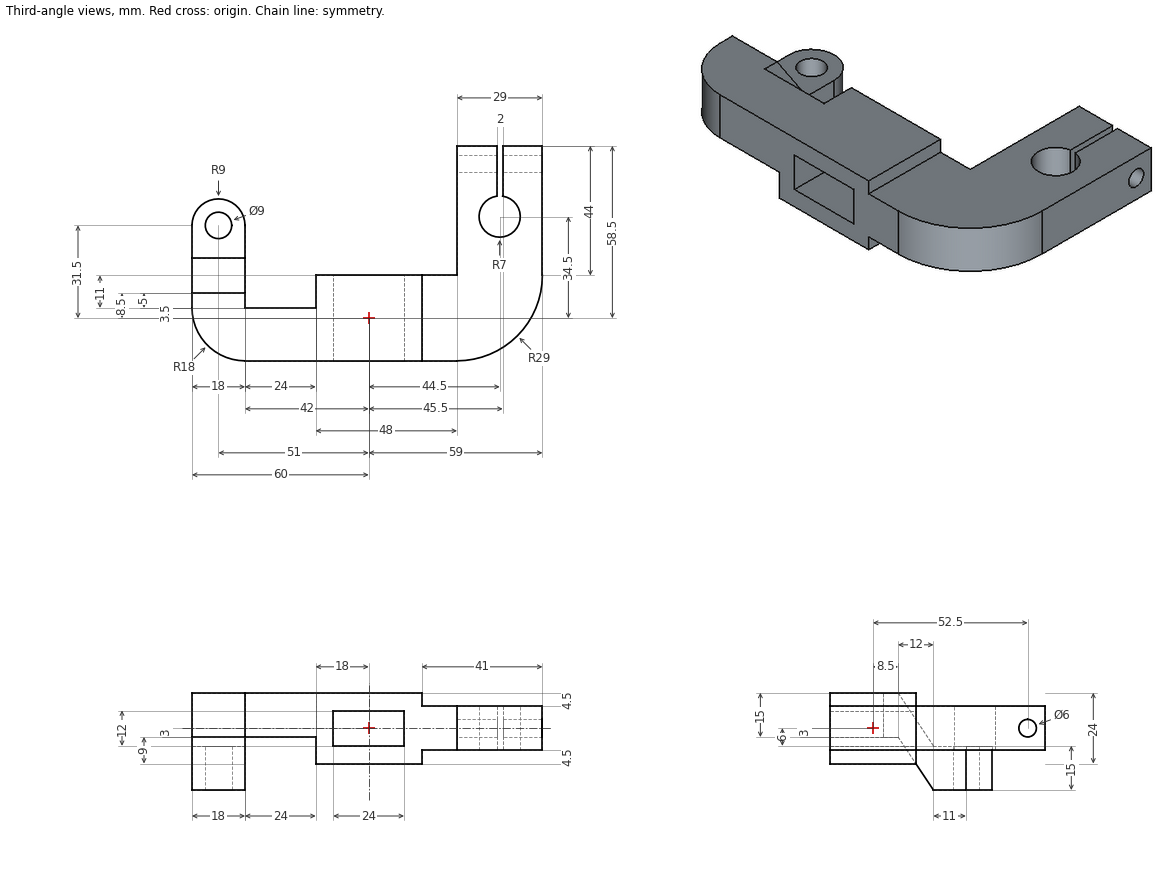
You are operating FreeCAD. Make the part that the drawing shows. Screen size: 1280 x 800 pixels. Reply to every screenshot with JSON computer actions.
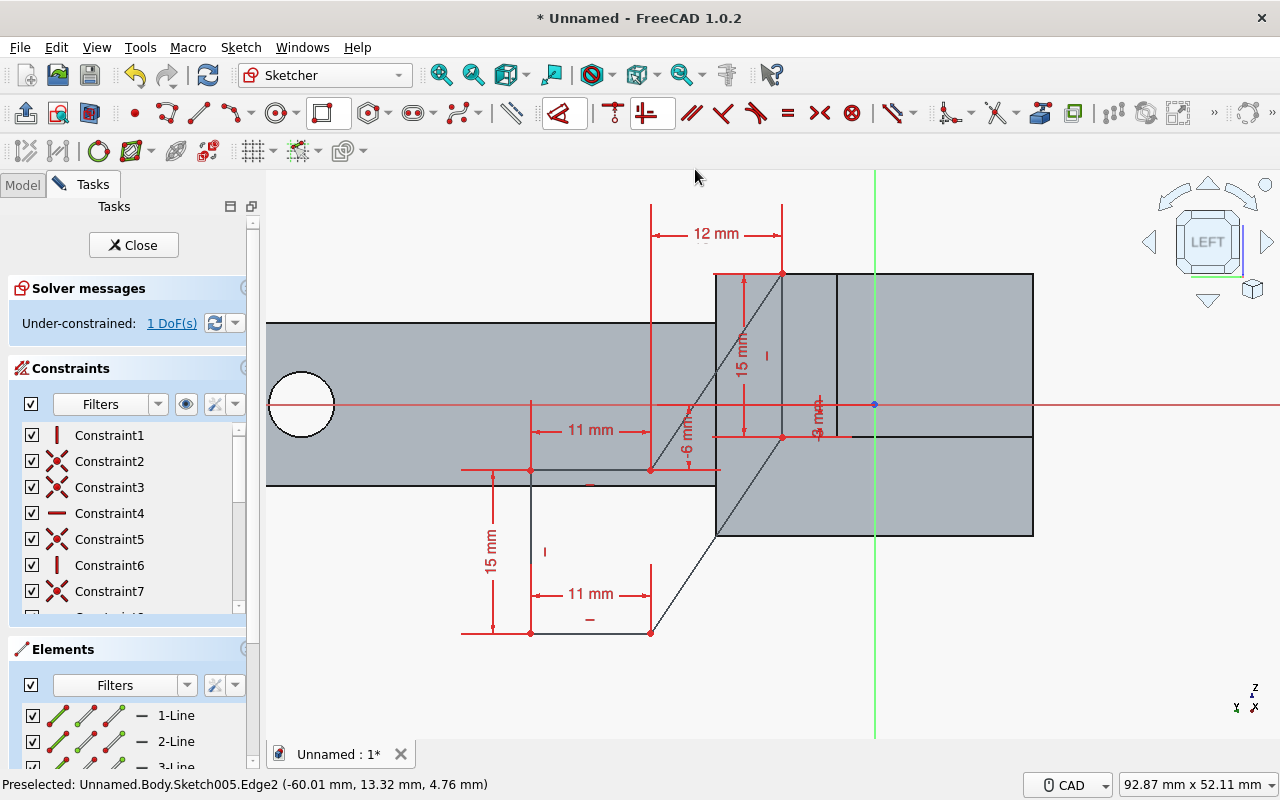
{"action": "left_click", "coordinate": [782, 437]}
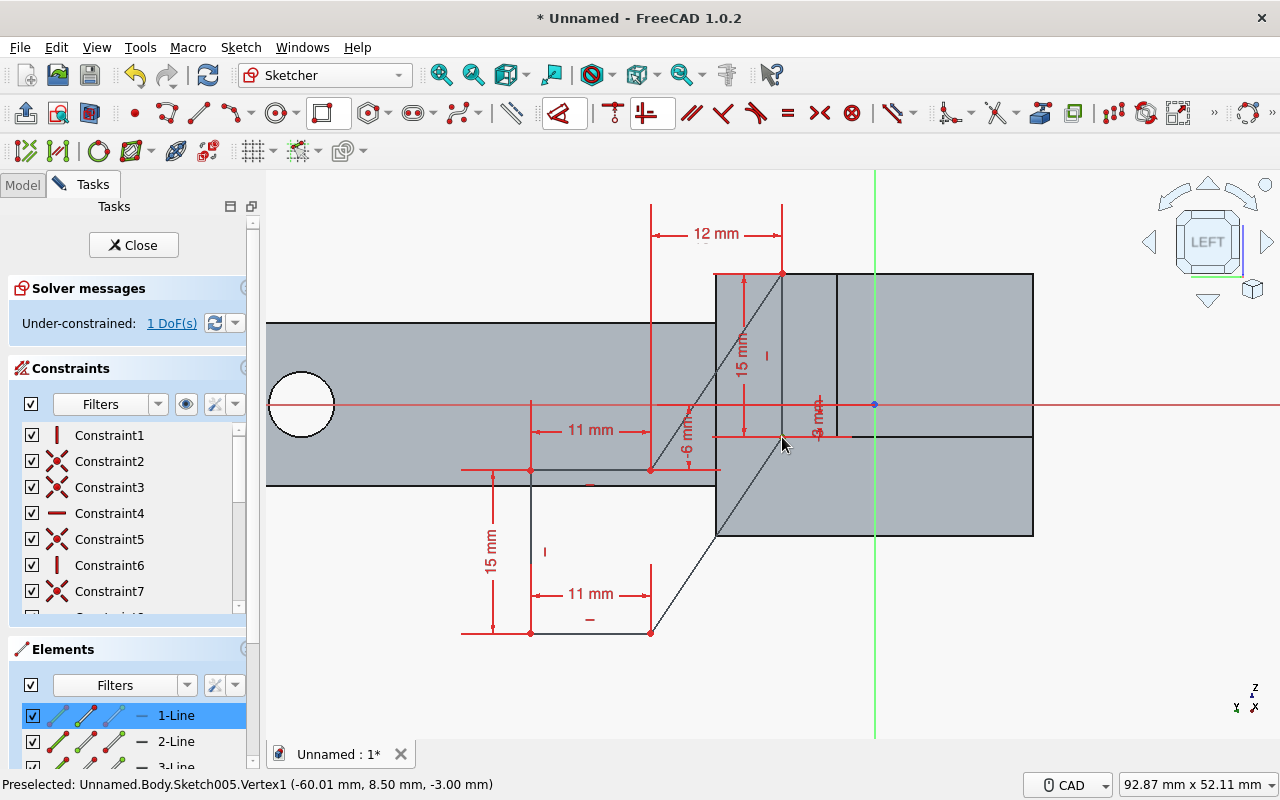
{"action": "left_click", "coordinate": [582, 114]}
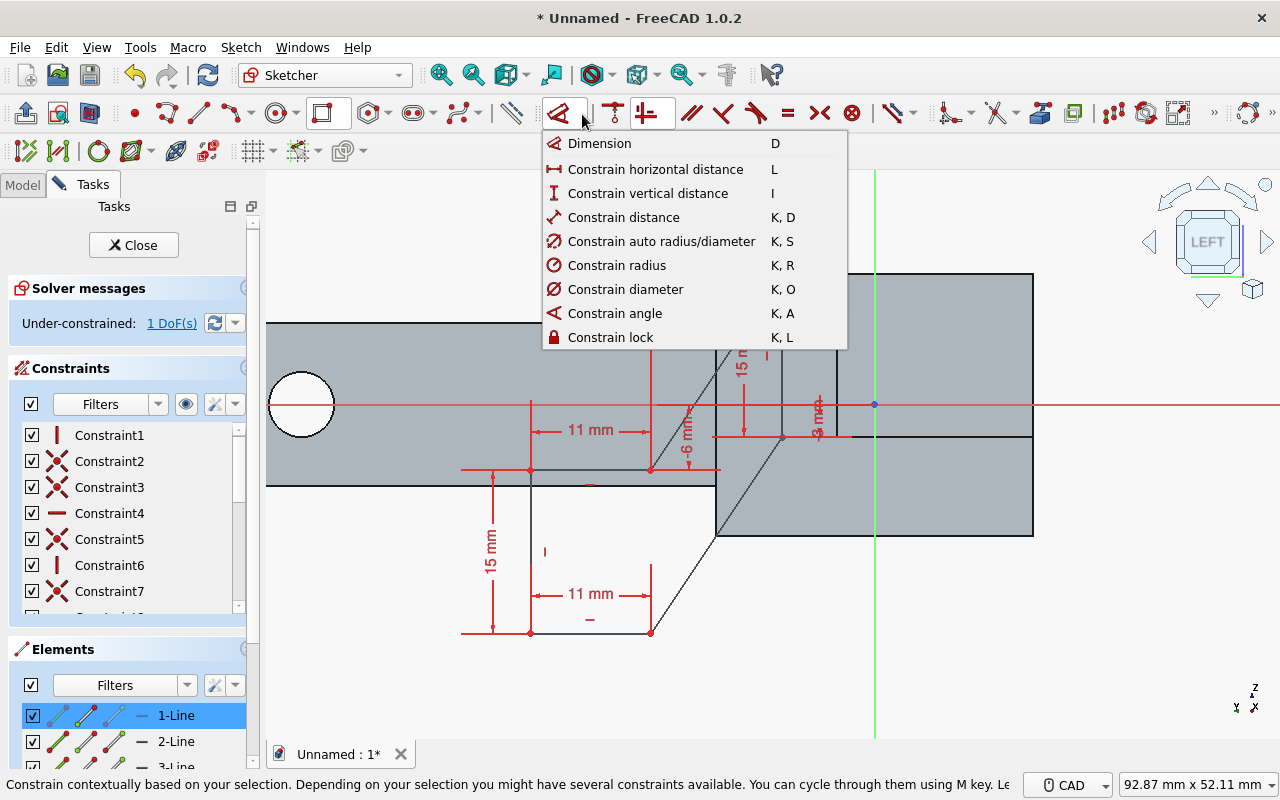
{"action": "left_click", "coordinate": [695, 169]}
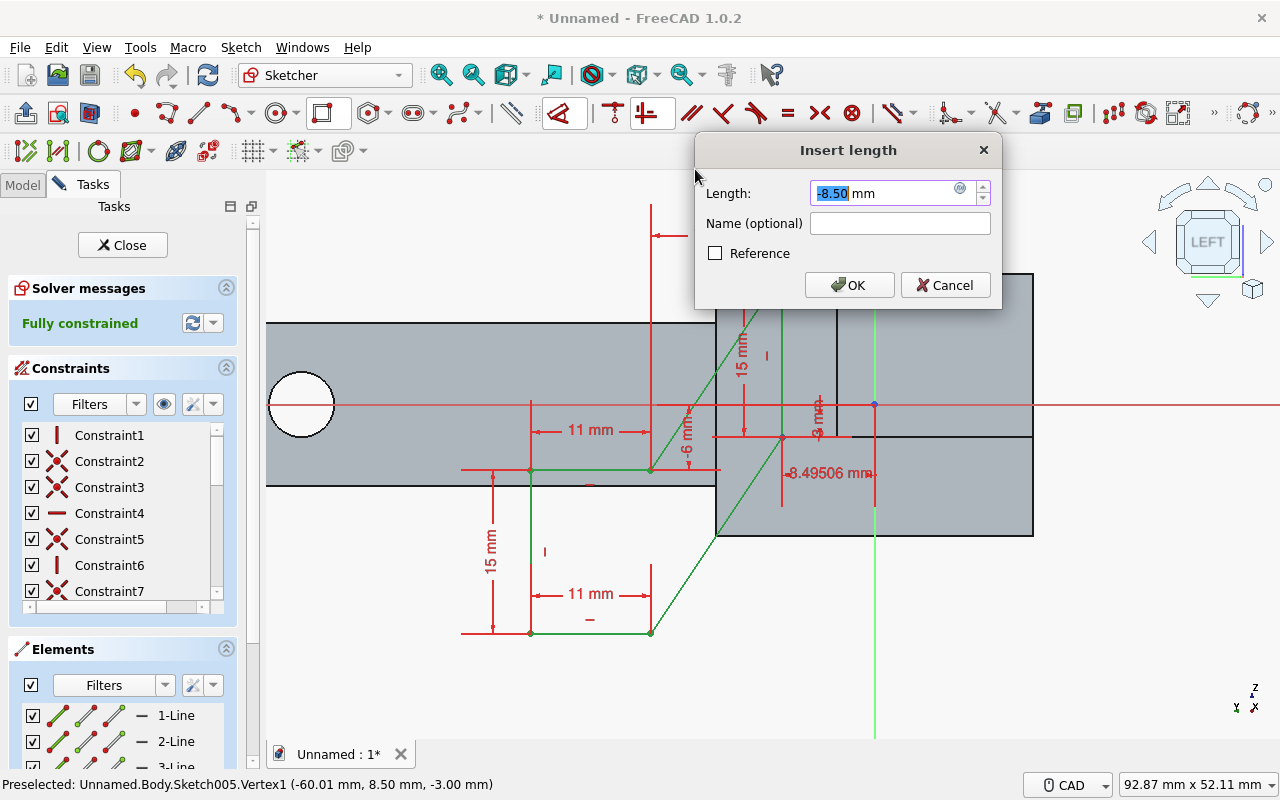
{"action": "type", "text": "-8.5"}
{"action": "key", "text": "Return"}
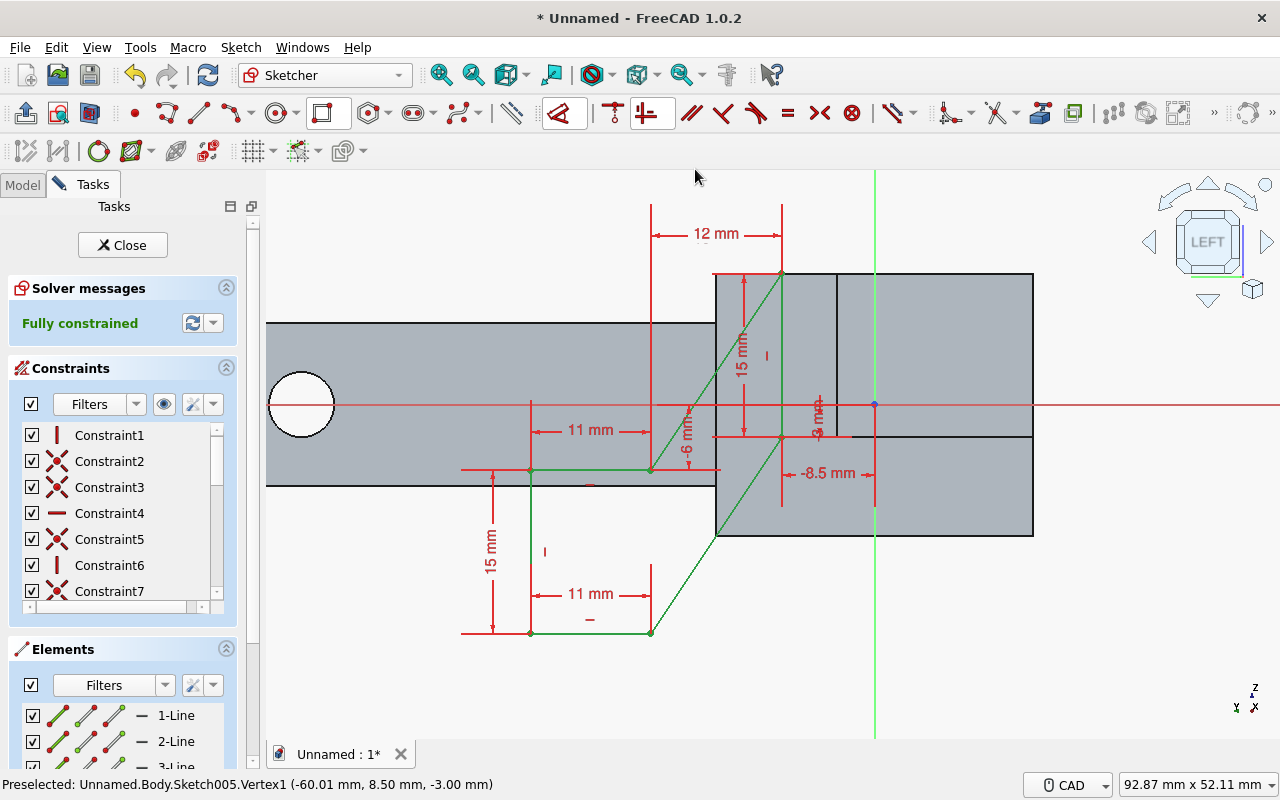
{"action": "left_click", "coordinate": [123, 245]}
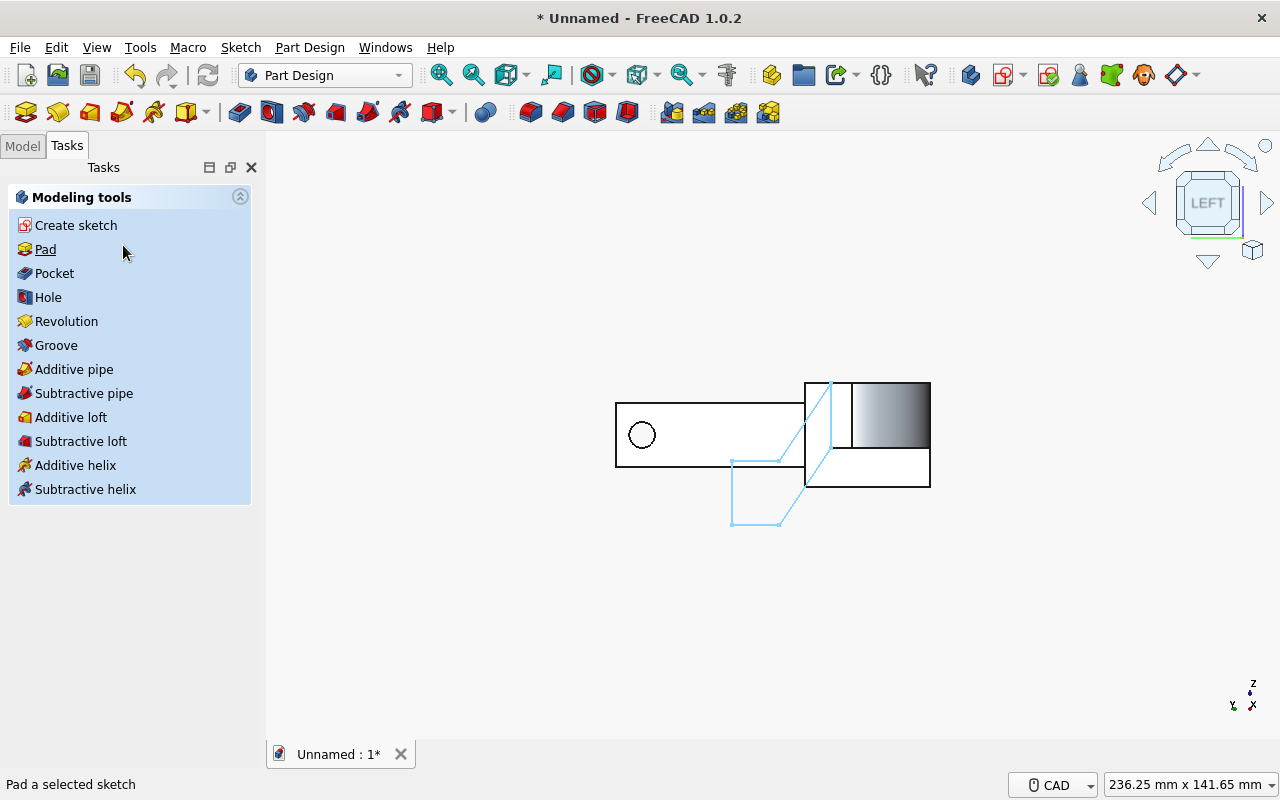
{"action": "left_click", "coordinate": [26, 112]}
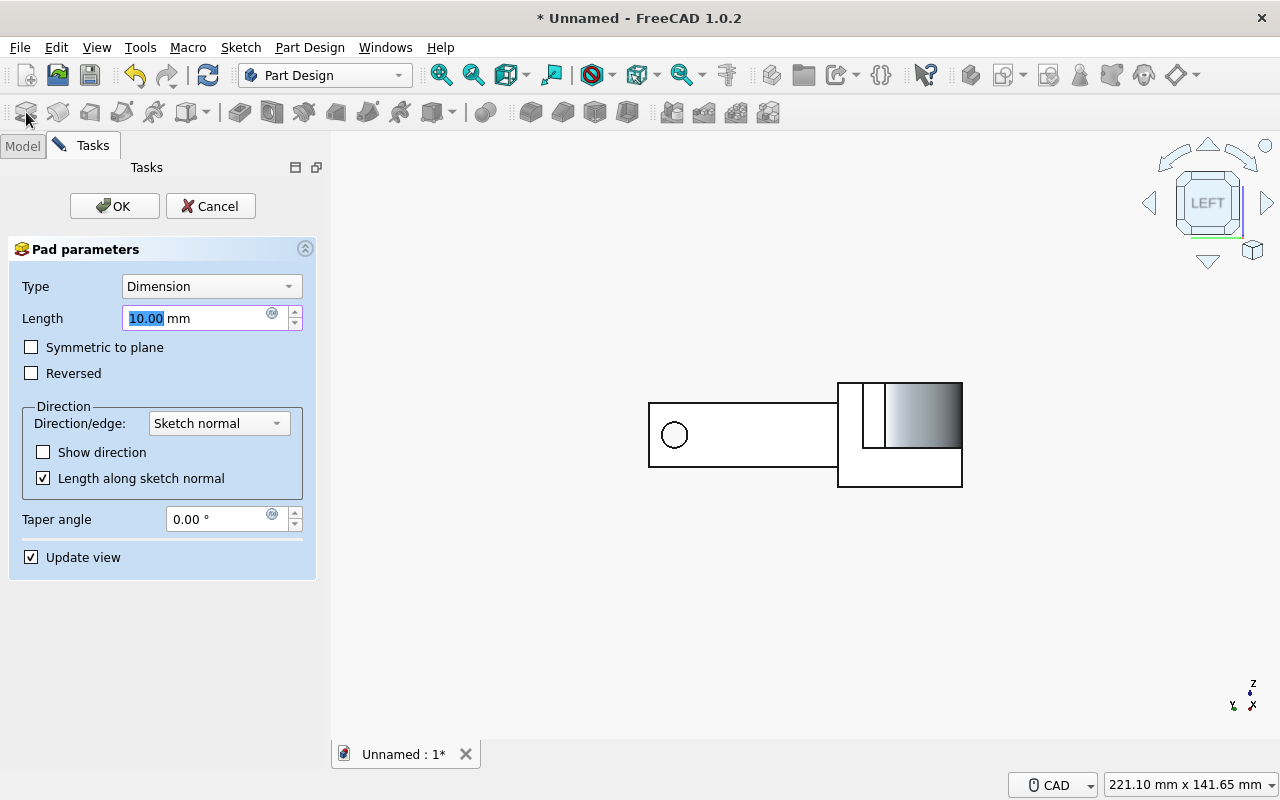
{"action": "type", "text": "18"}
{"action": "key", "text": "Tab"}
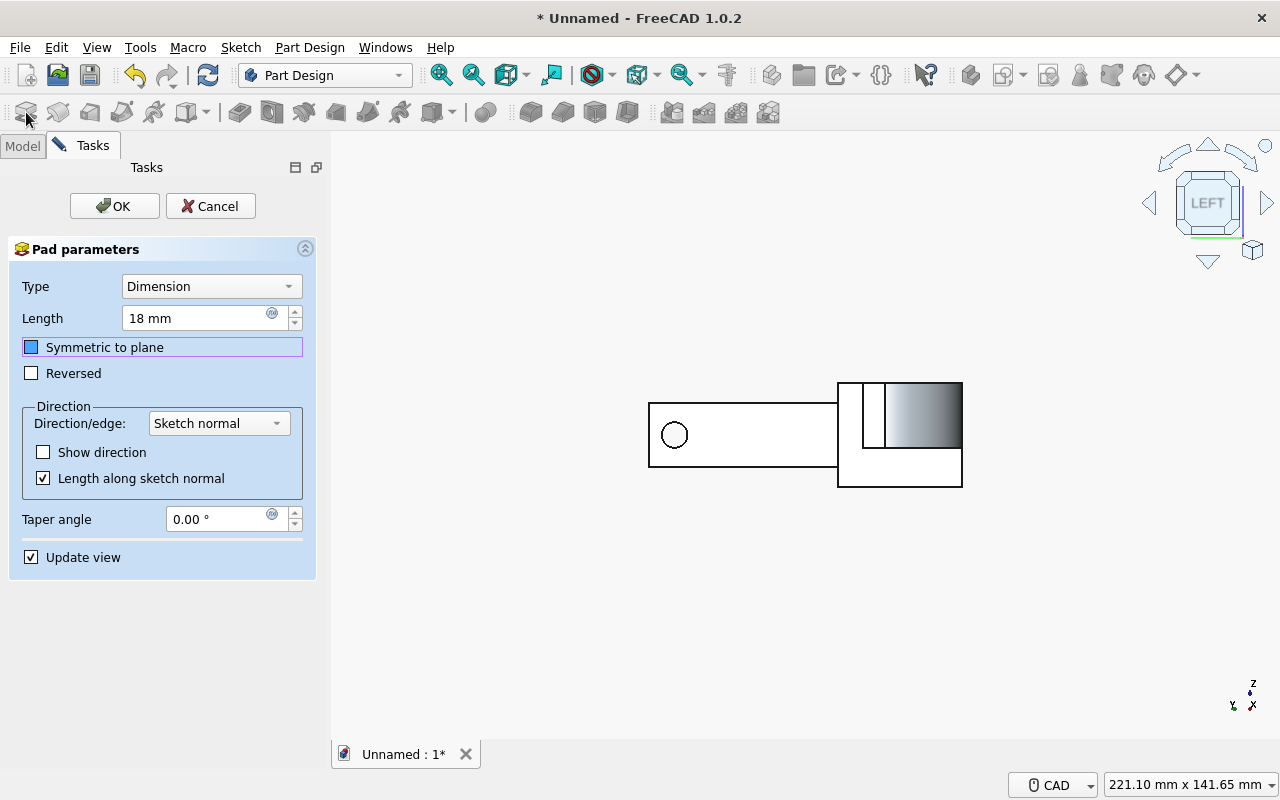
{"action": "left_click", "coordinate": [30, 373]}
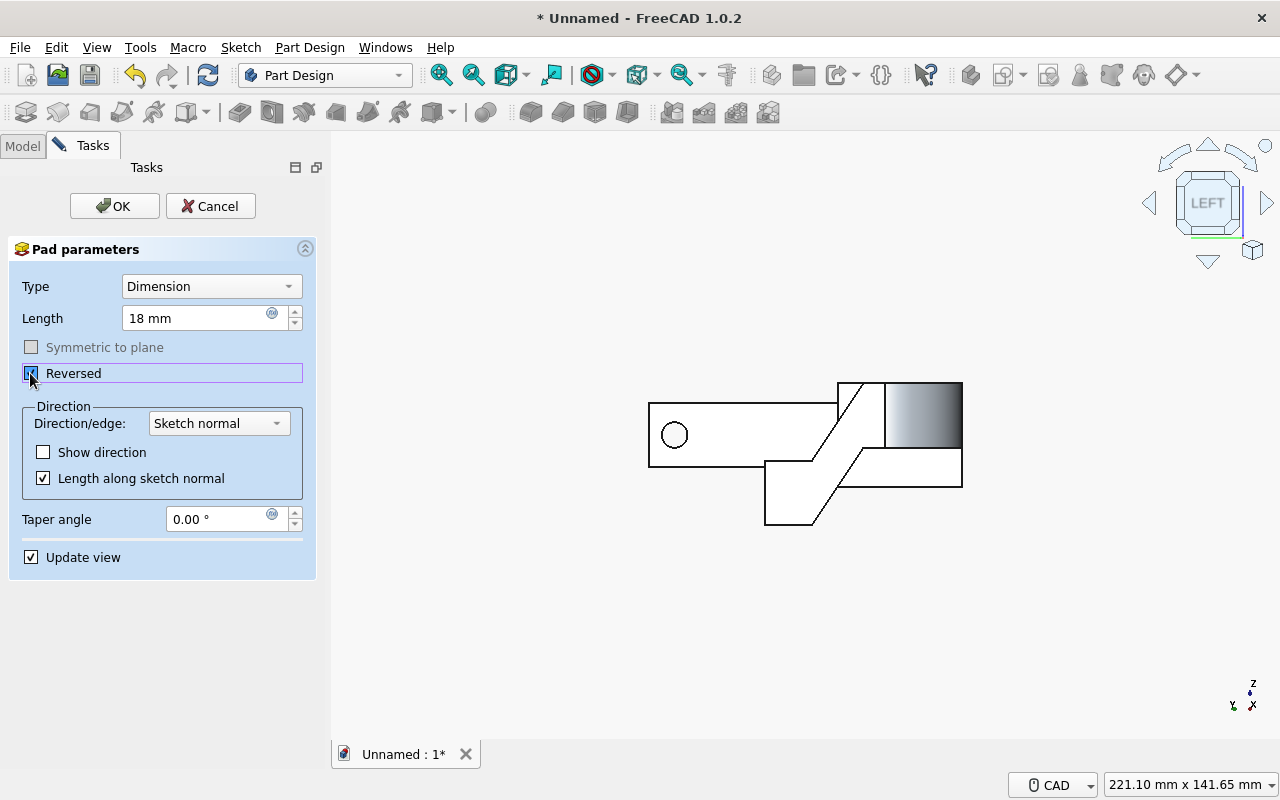
{"action": "left_click", "coordinate": [115, 206]}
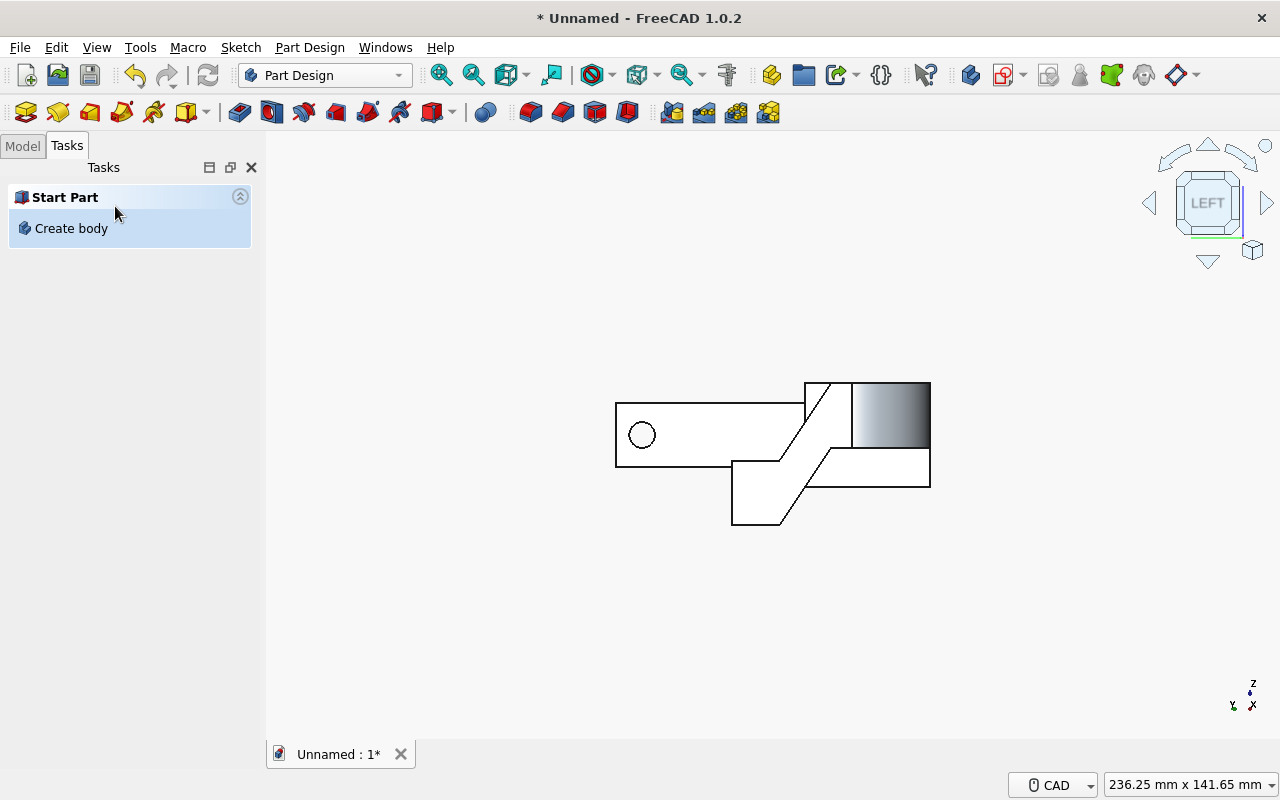
{"action": "left_click", "coordinate": [442, 76]}